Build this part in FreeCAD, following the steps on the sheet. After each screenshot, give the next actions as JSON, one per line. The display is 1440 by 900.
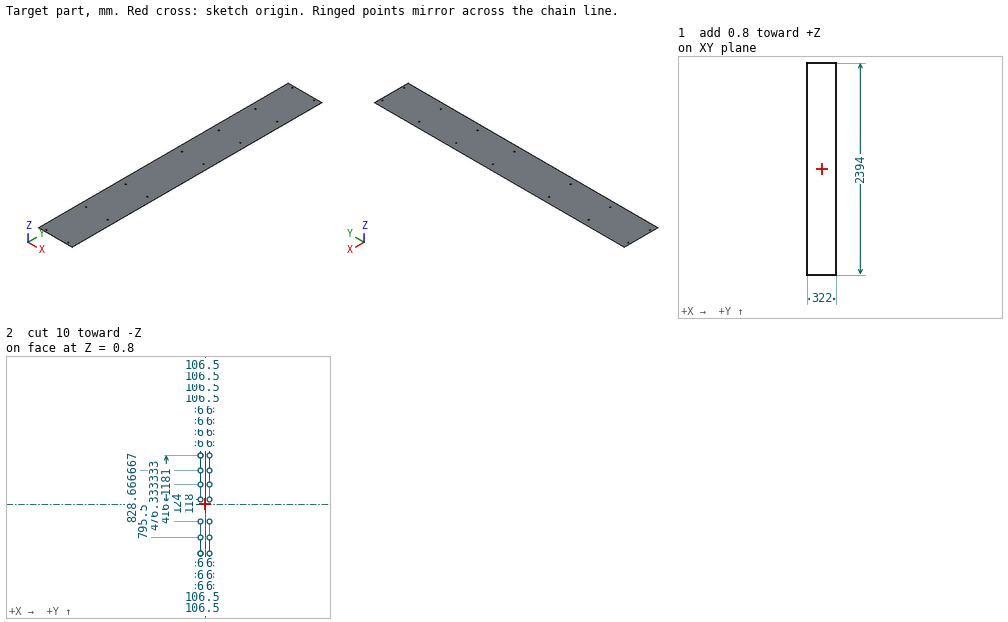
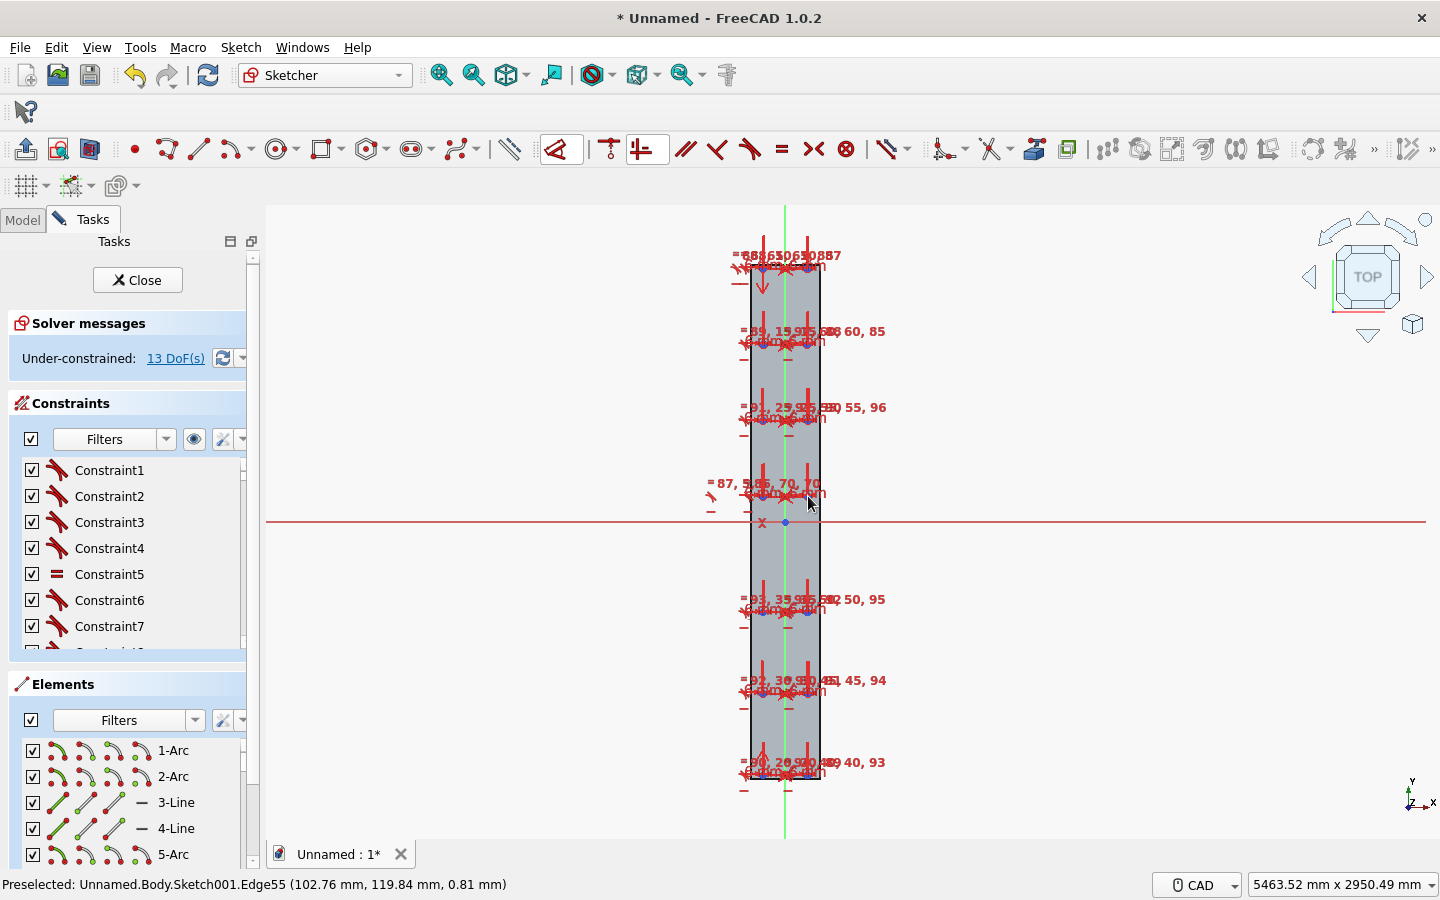
{"action": "scroll", "coordinate": [762, 496], "scroll_direction": "up", "scroll_amount": 13}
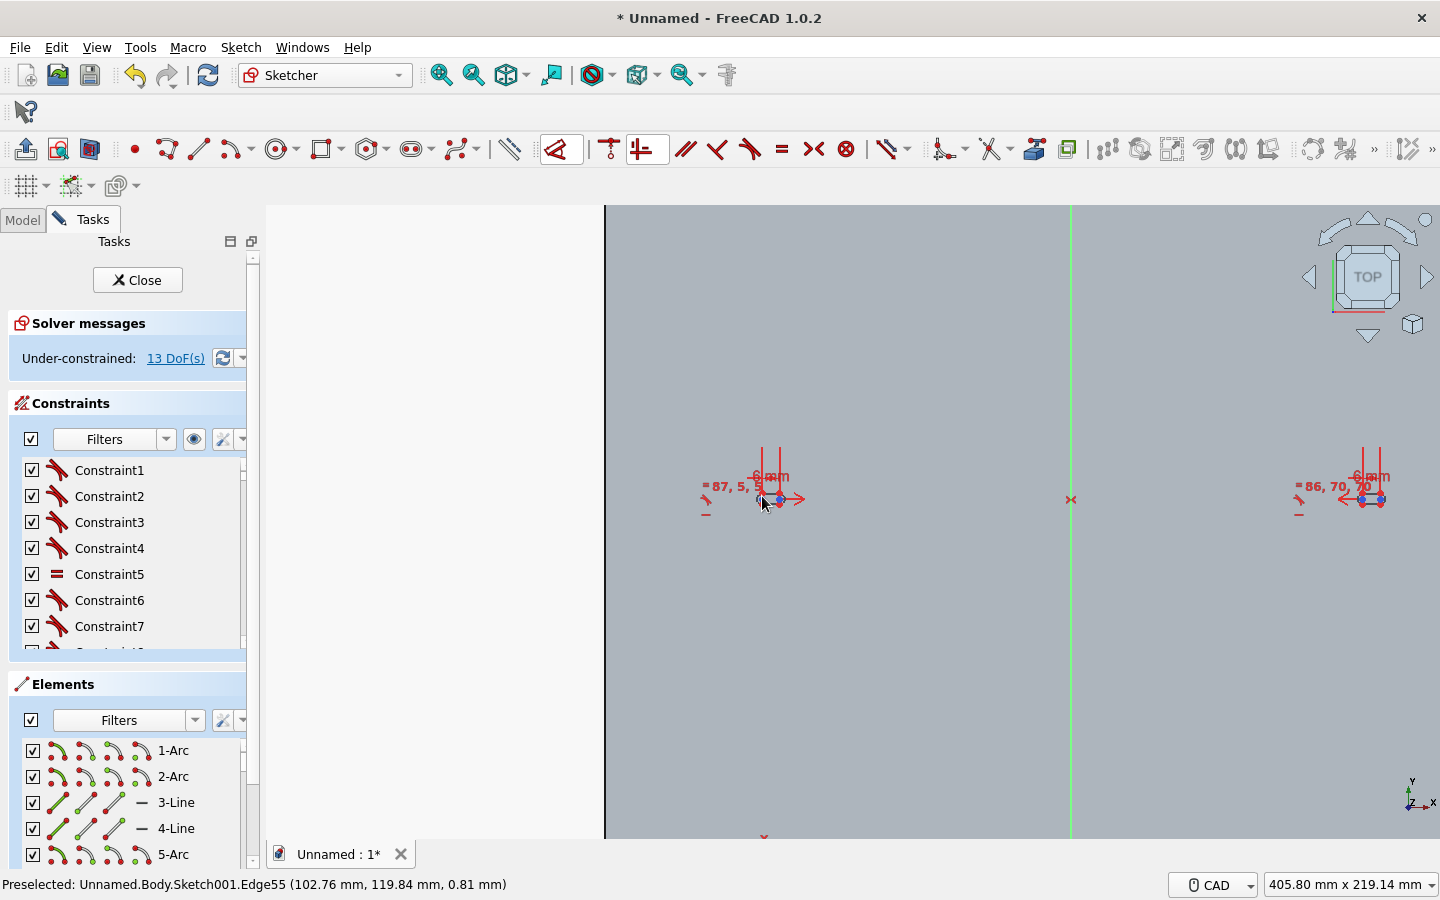
{"action": "left_click", "coordinate": [760, 492]}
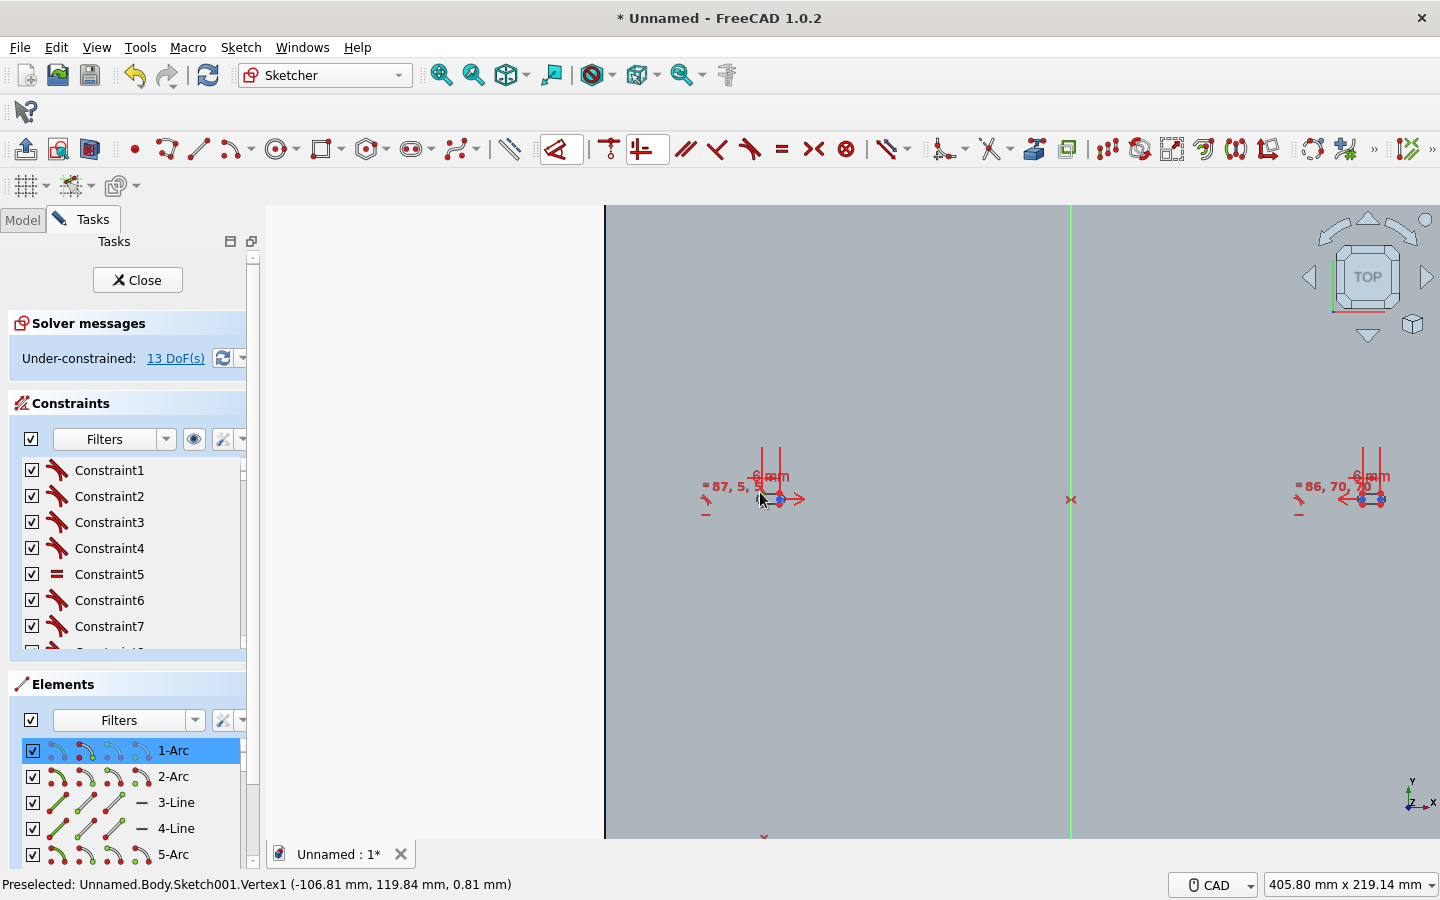
{"action": "key", "text": "i"}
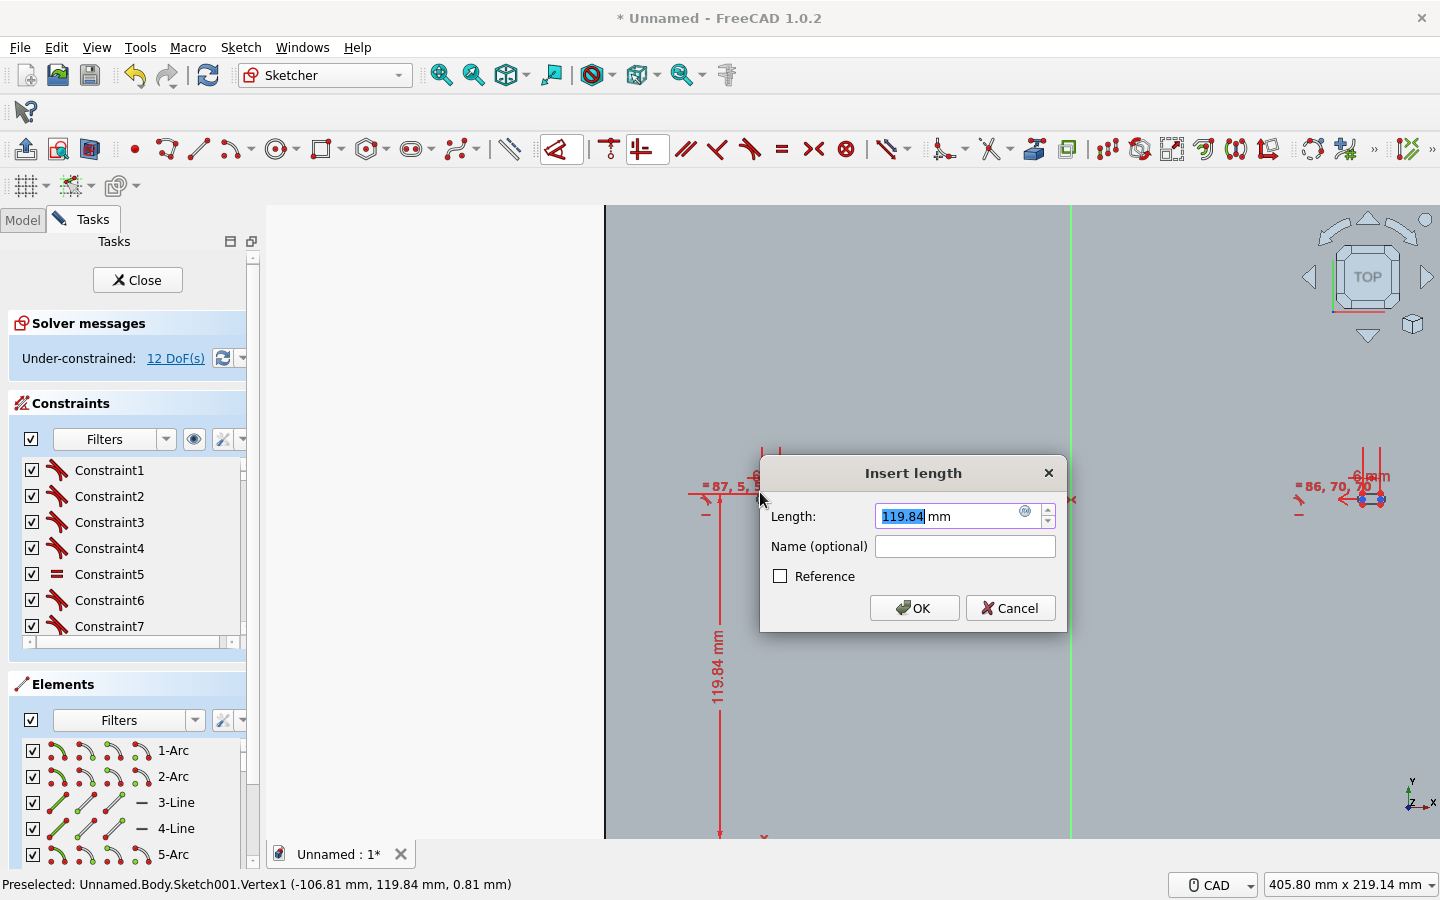
{"action": "type", "text": "124"}
{"action": "key", "text": "Return"}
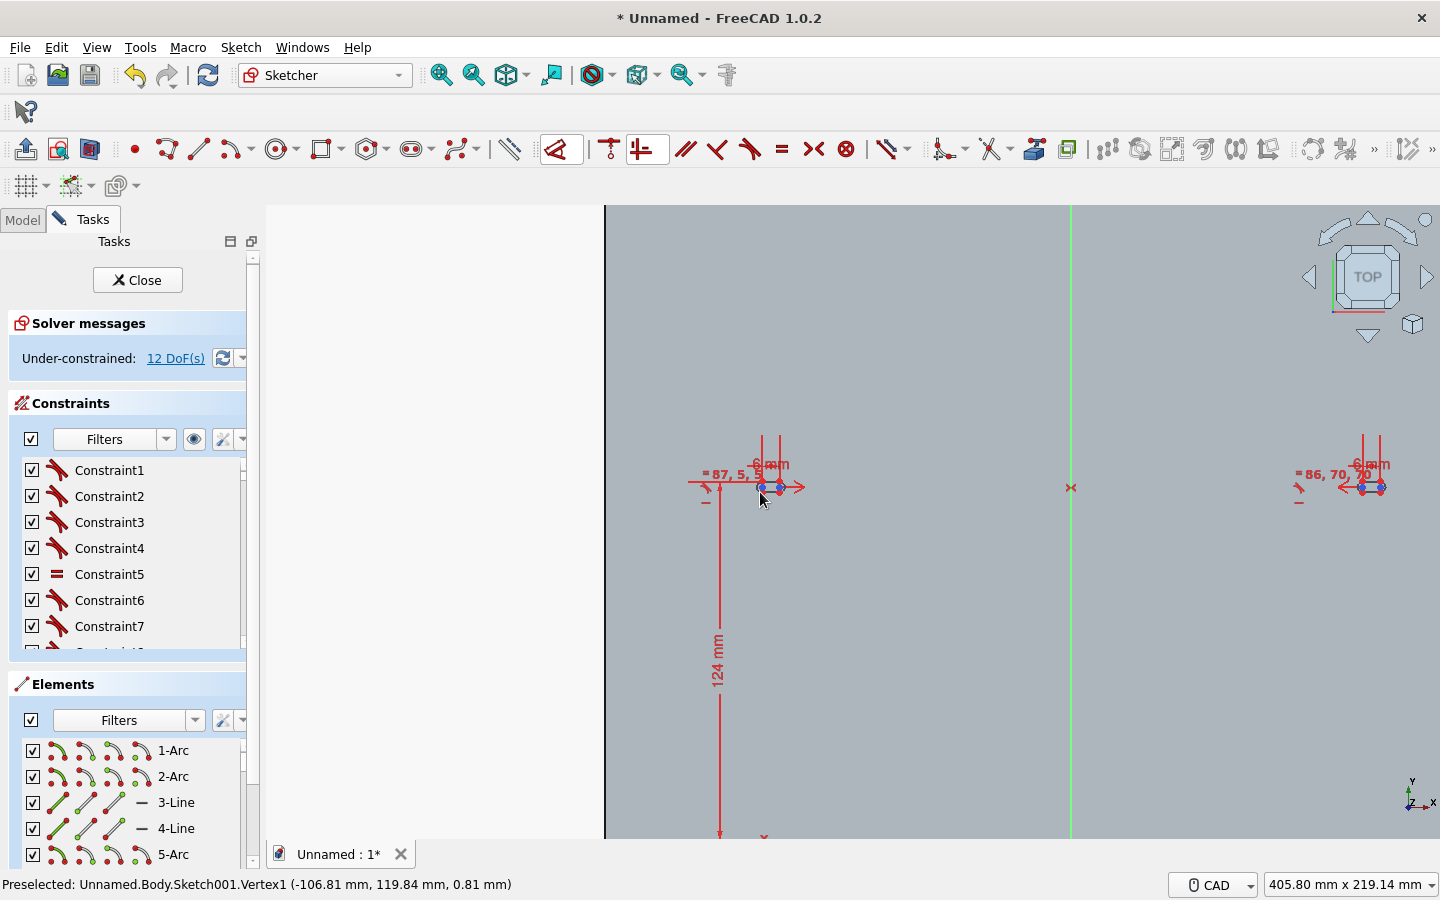
{"action": "left_click", "coordinate": [762, 492]}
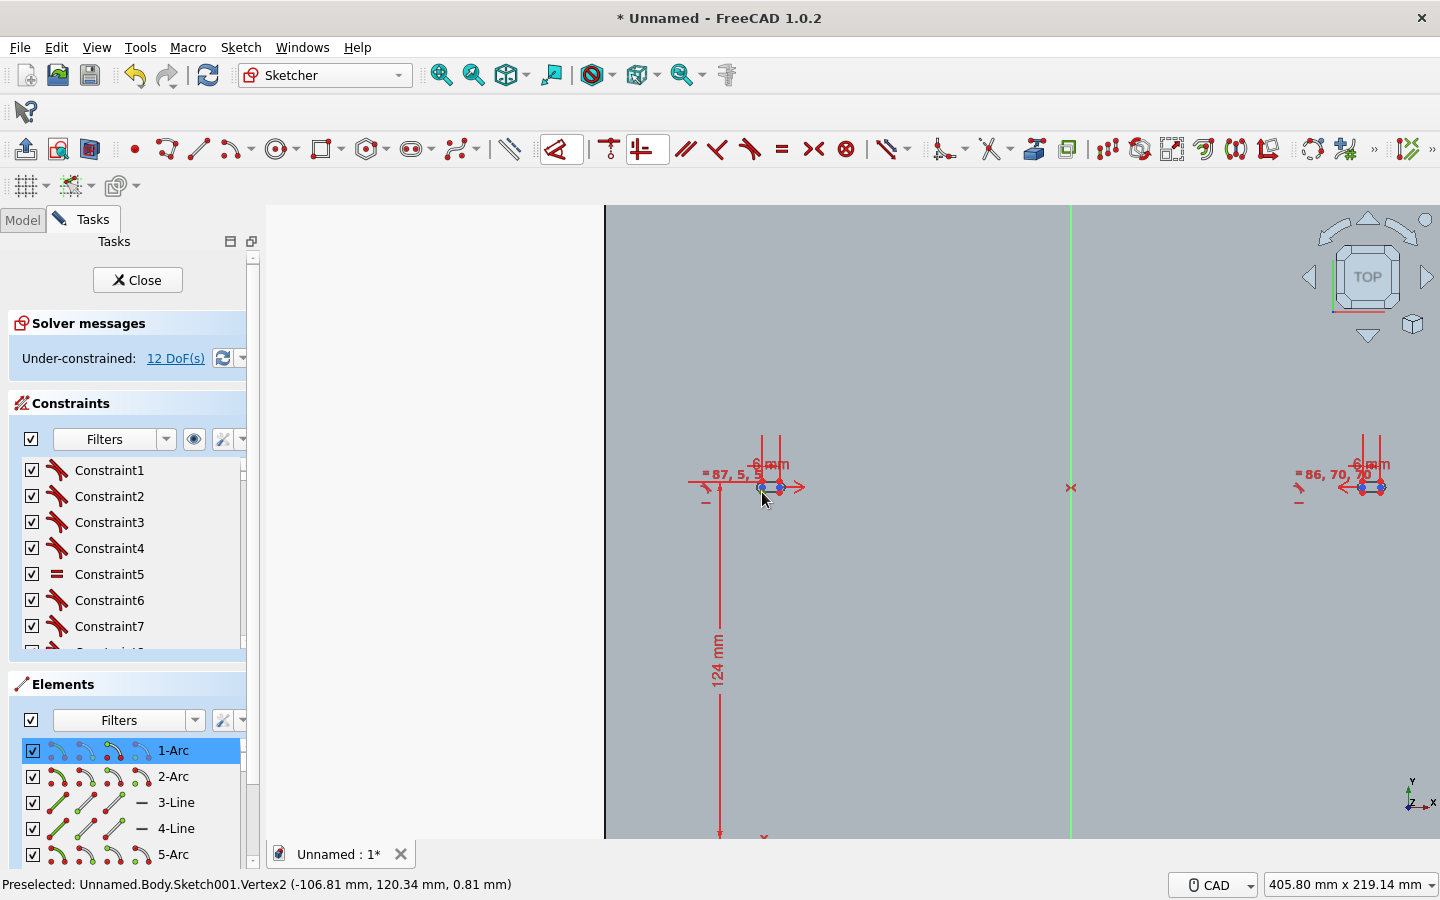
{"action": "key", "text": "i"}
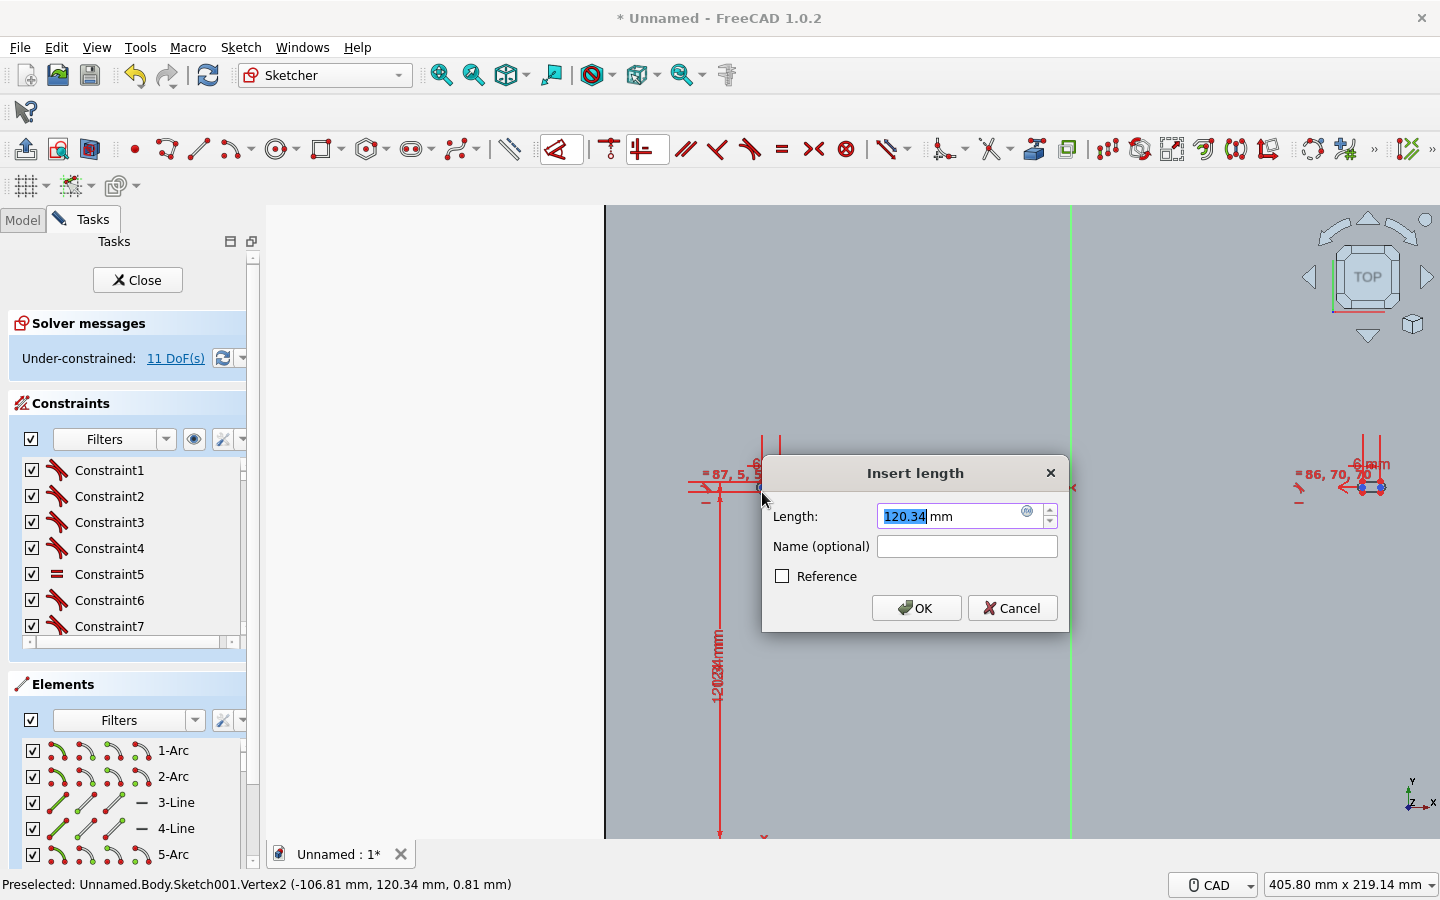
{"action": "type", "text": "118"}
{"action": "key", "text": "Return"}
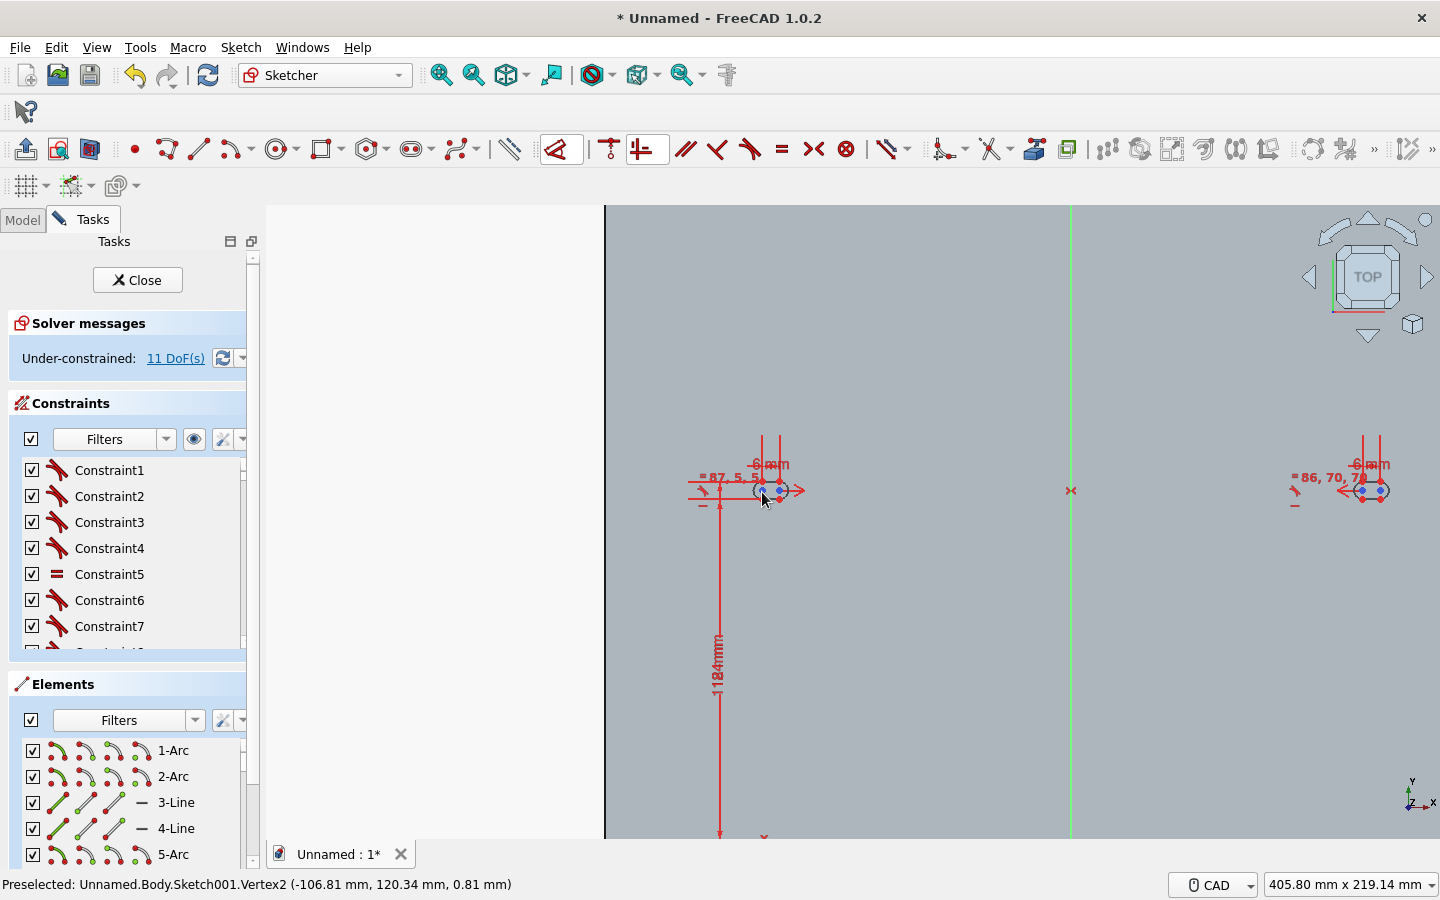
{"action": "scroll", "coordinate": [766, 501], "scroll_direction": "down", "scroll_amount": 14}